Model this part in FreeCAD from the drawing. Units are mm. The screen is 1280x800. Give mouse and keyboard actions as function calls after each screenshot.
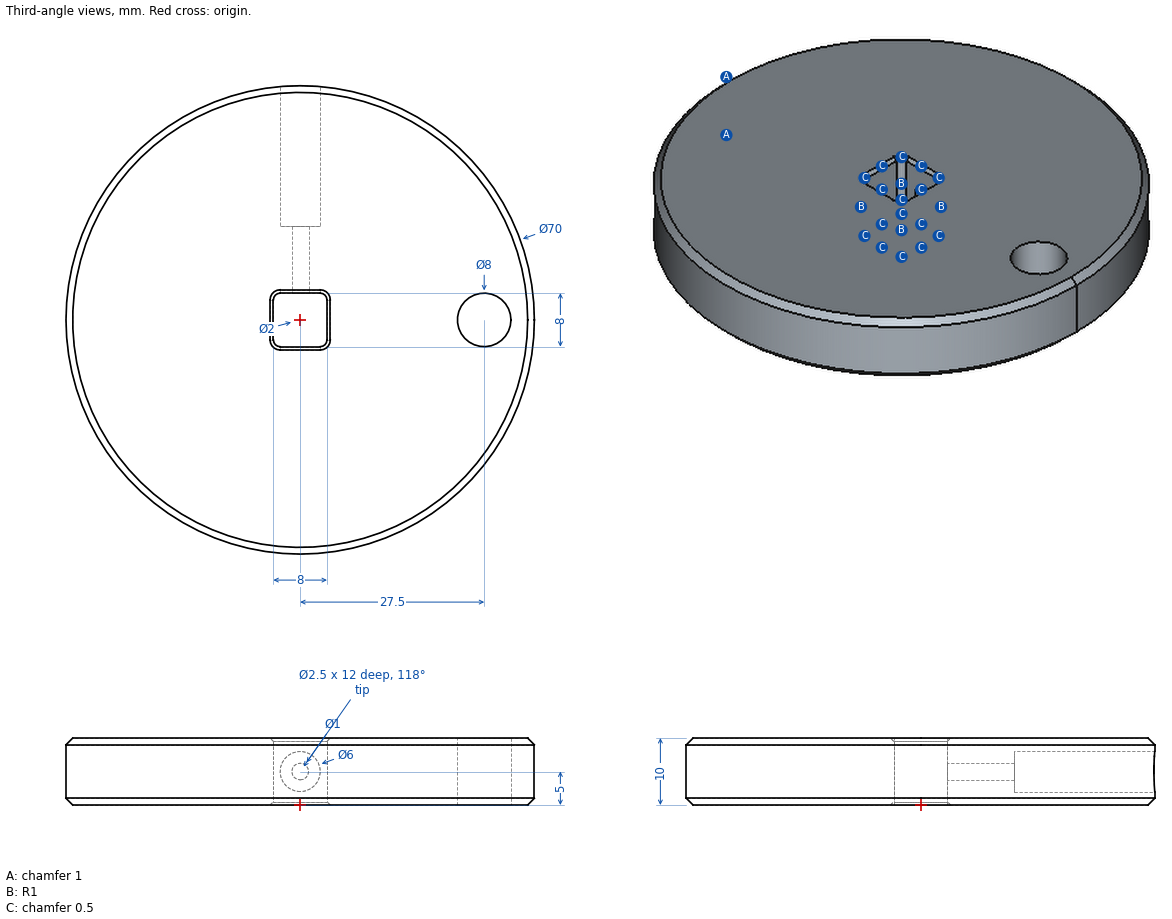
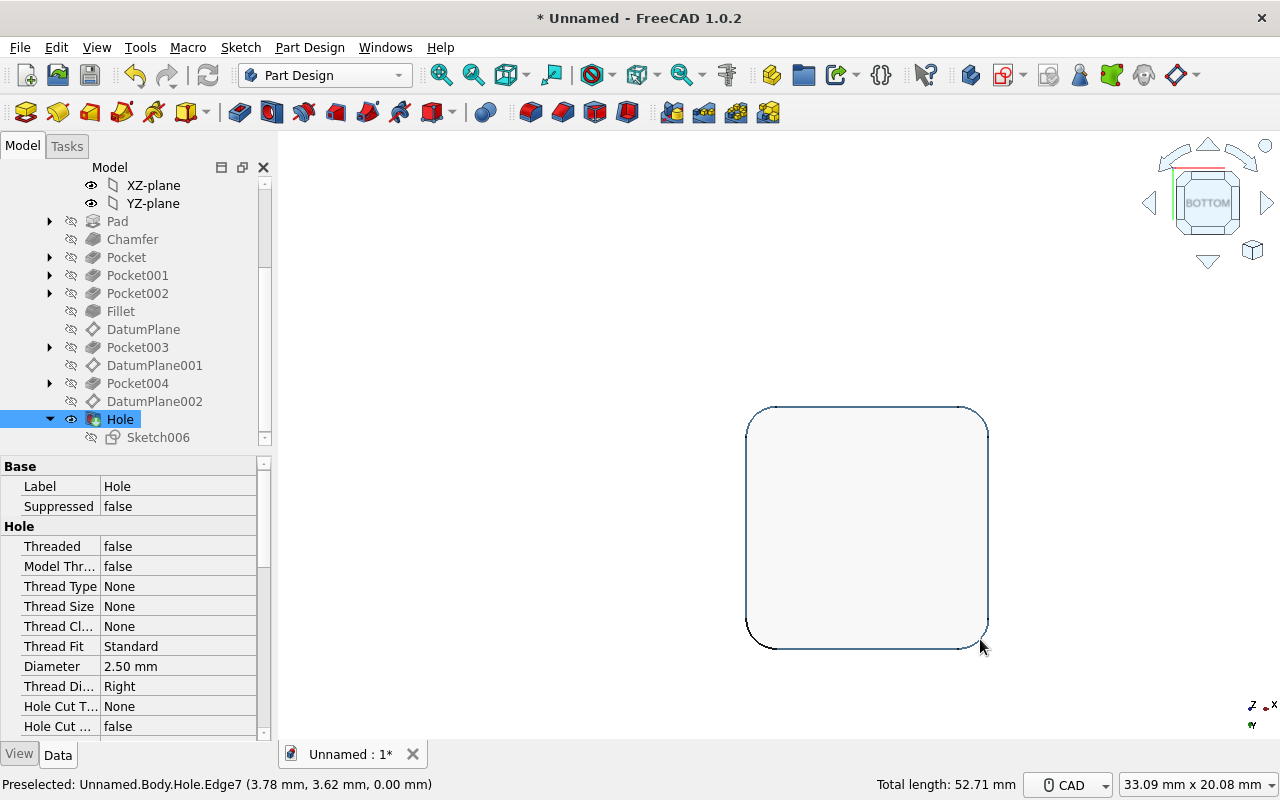
click(759, 642, ctrl)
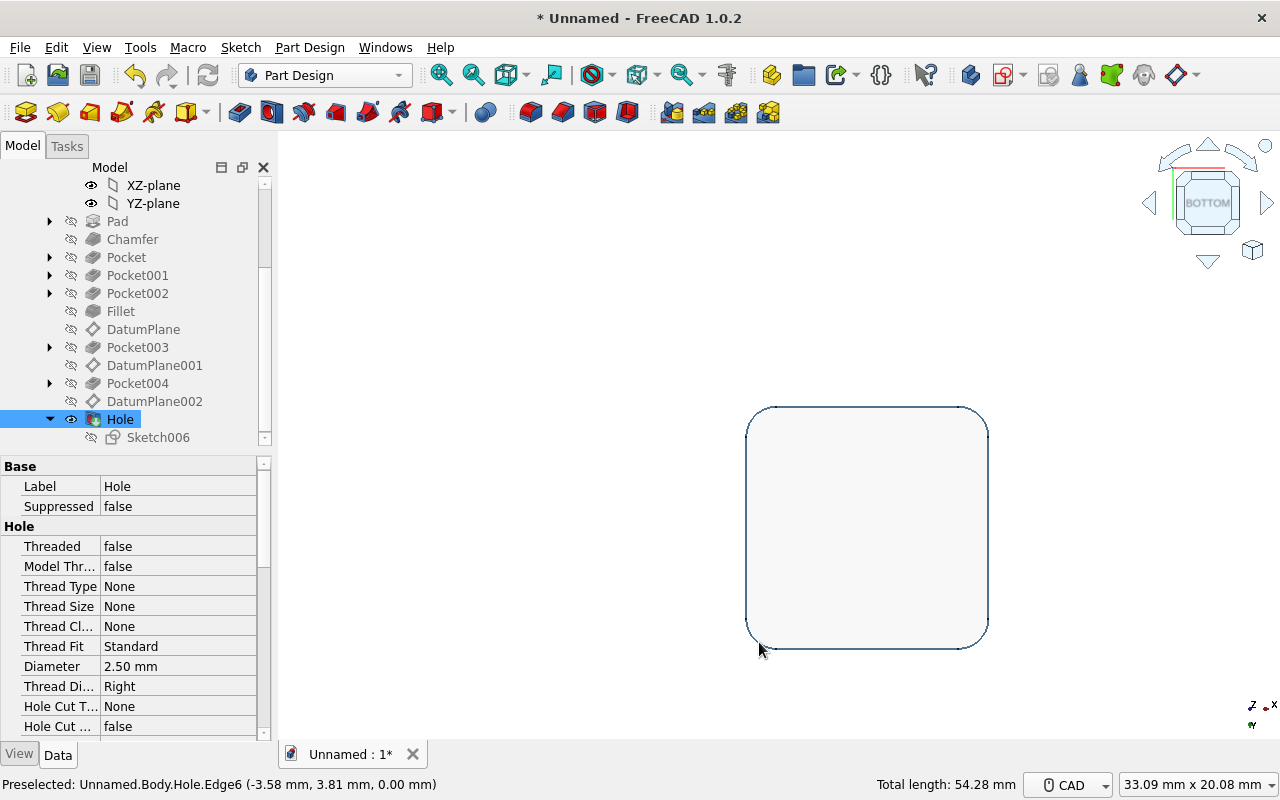
key(v)
key(f)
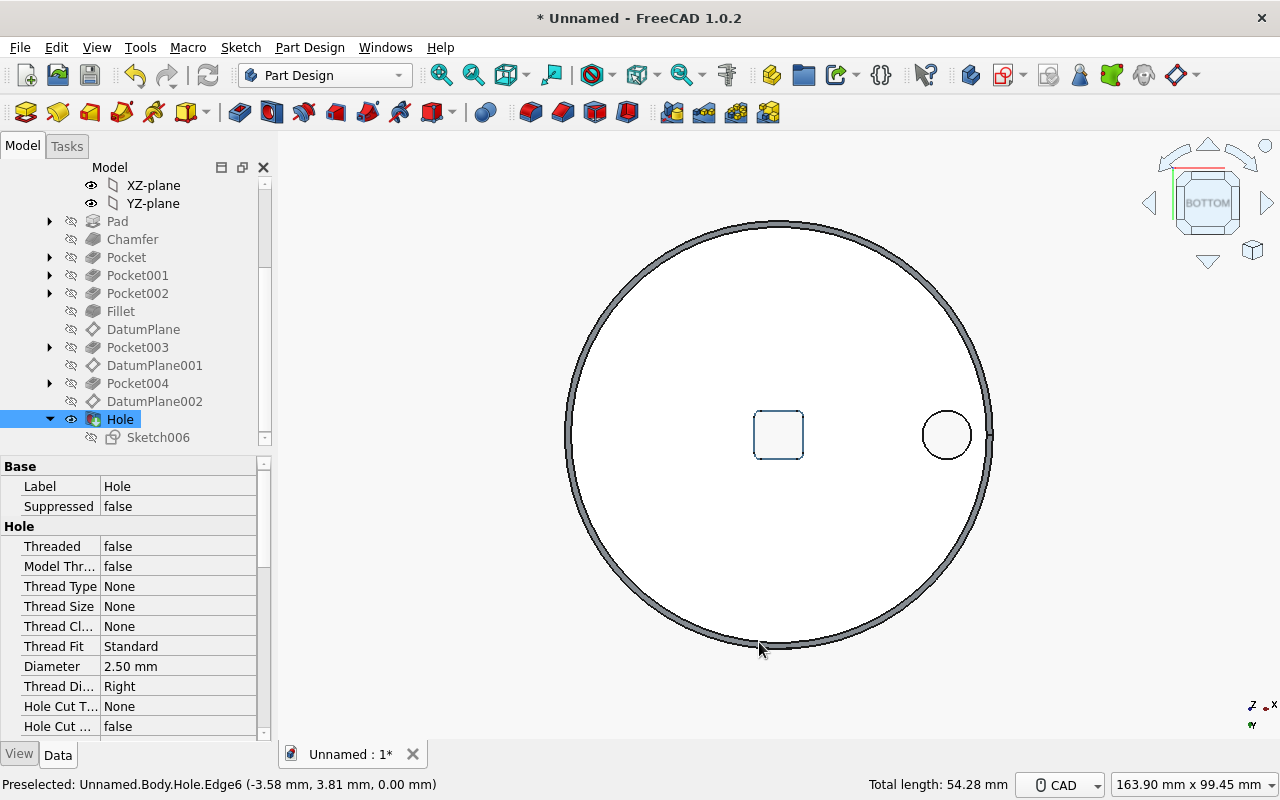
key(4)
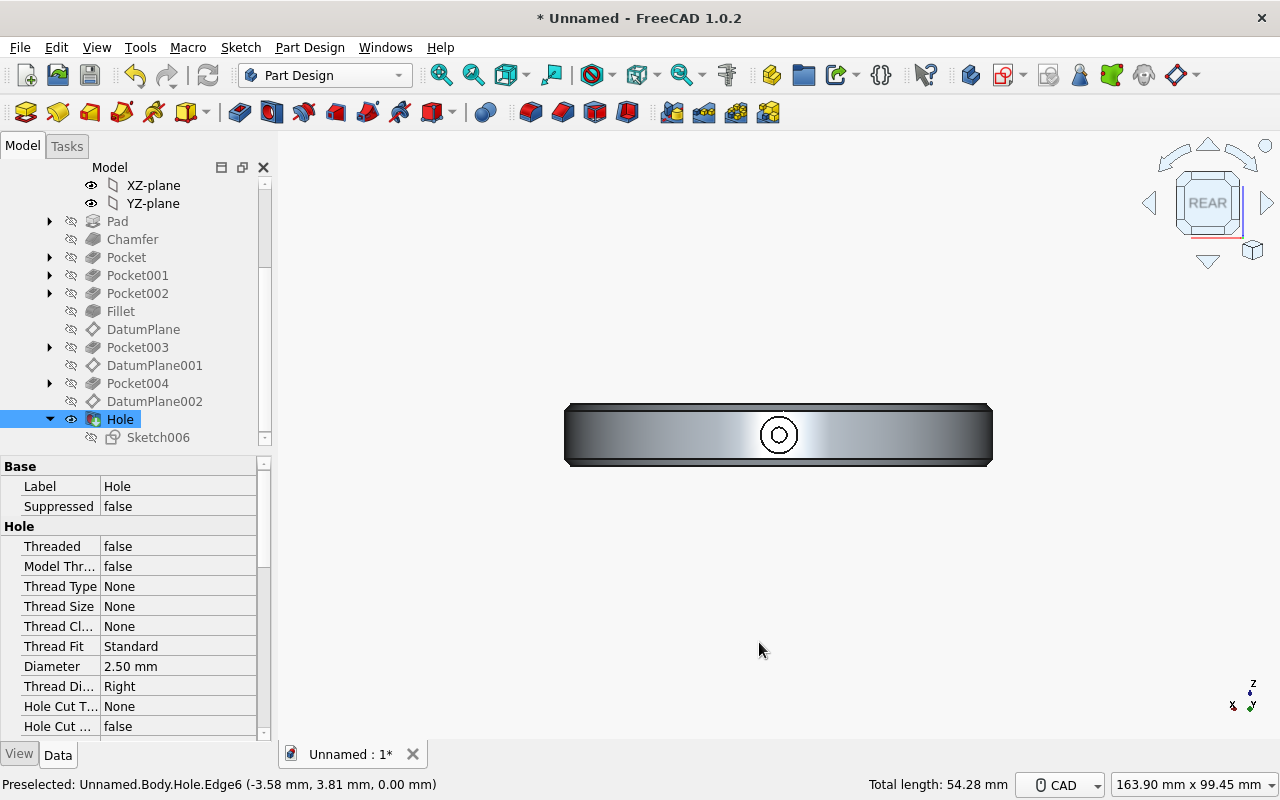
key(v)
key(f)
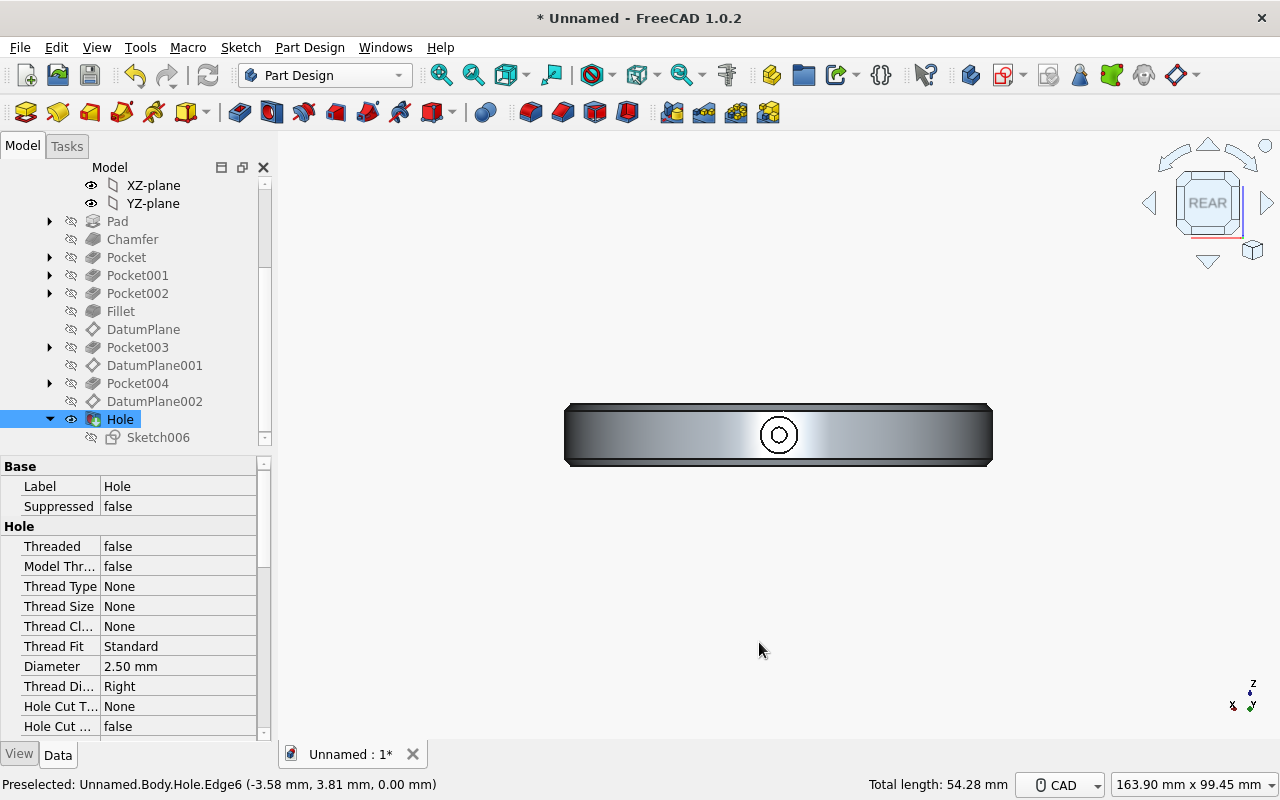
scroll(802, 403, up, 8)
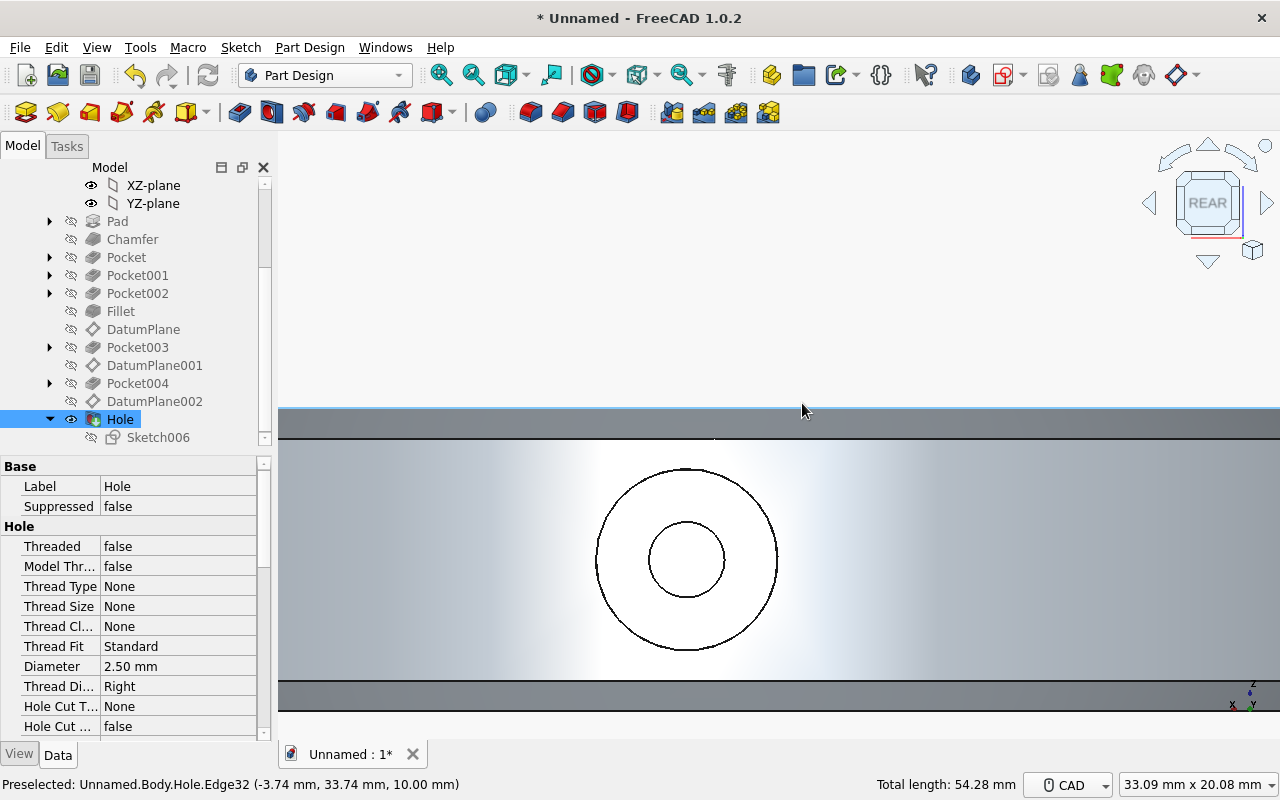
click(442, 76)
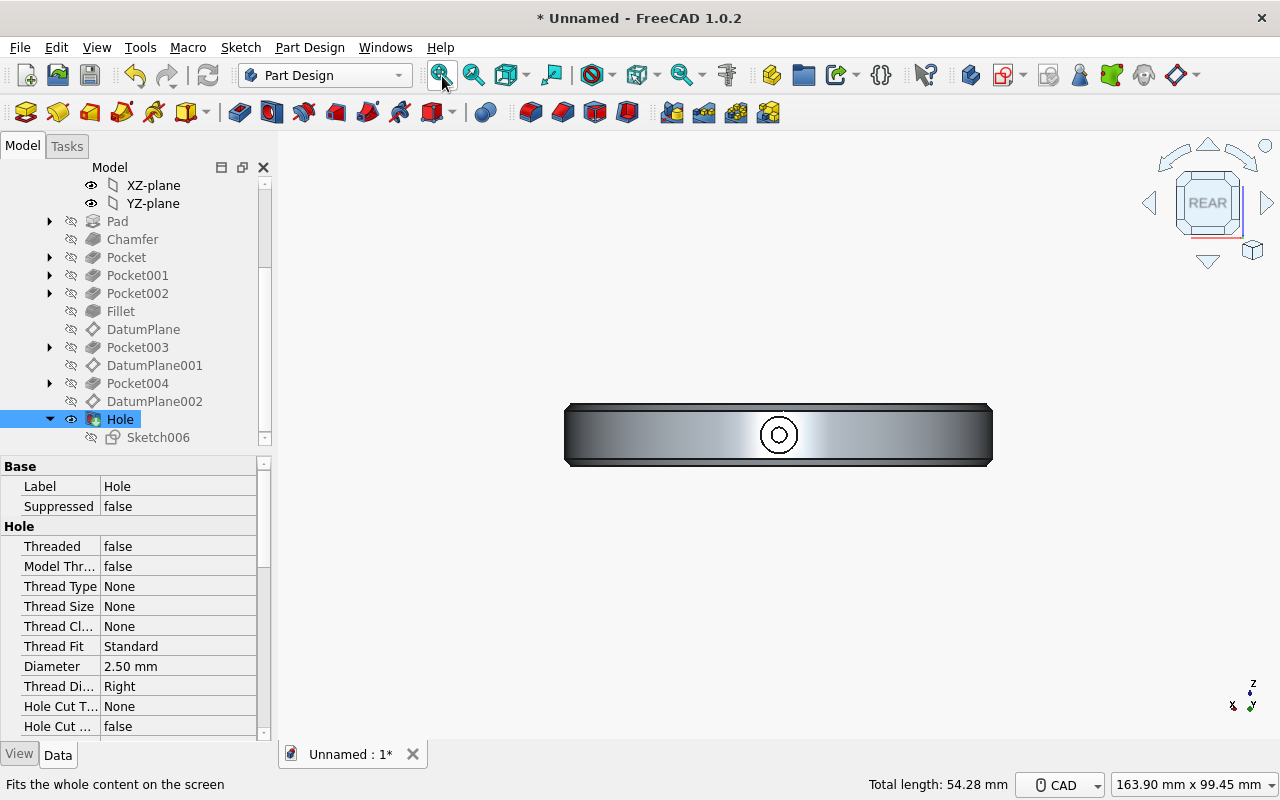
key(6)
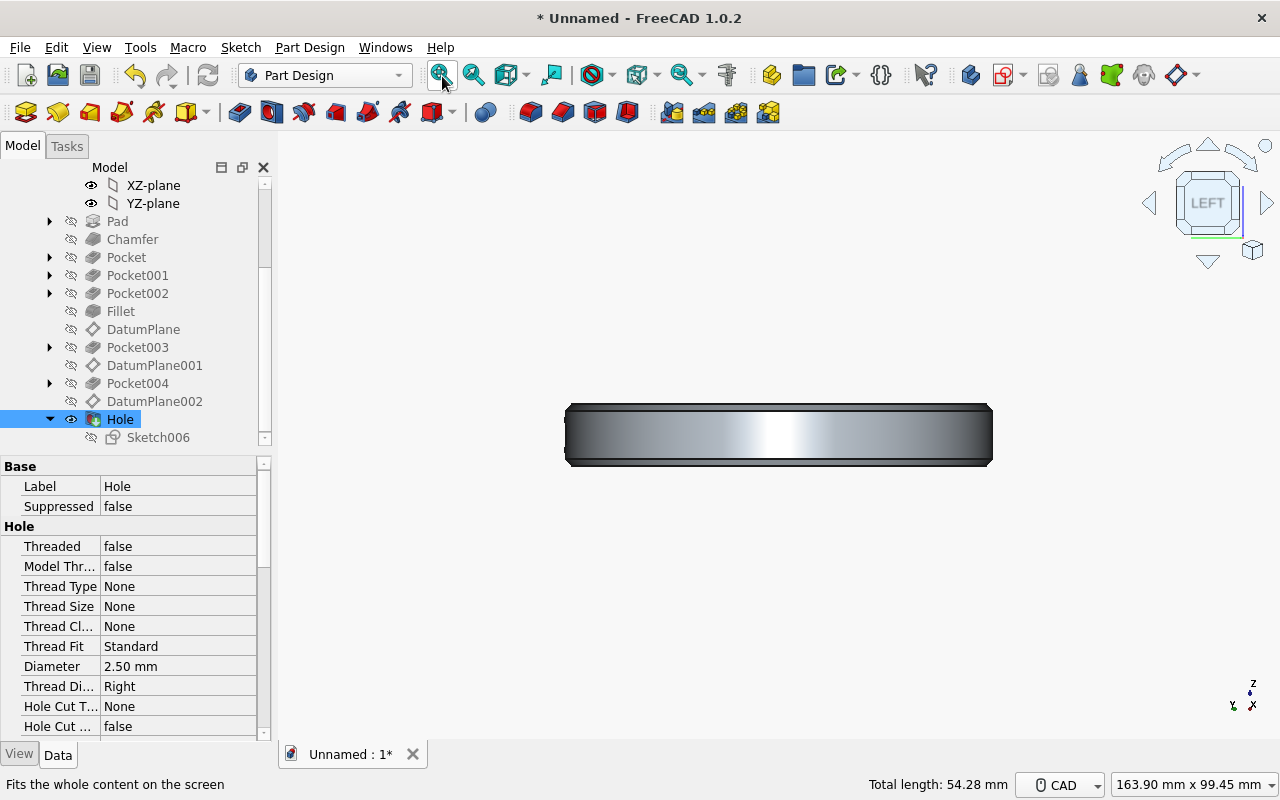
key(v)
key(f)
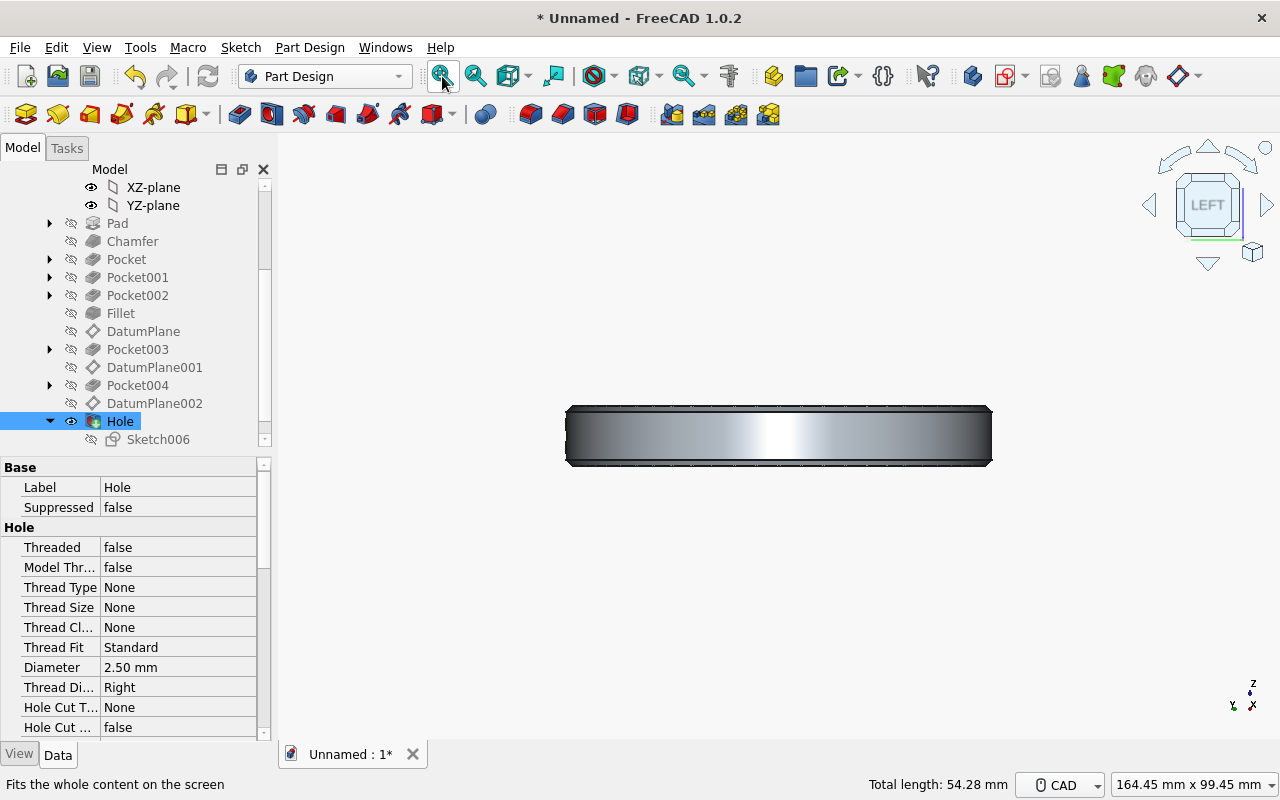
scroll(802, 405, up, 8)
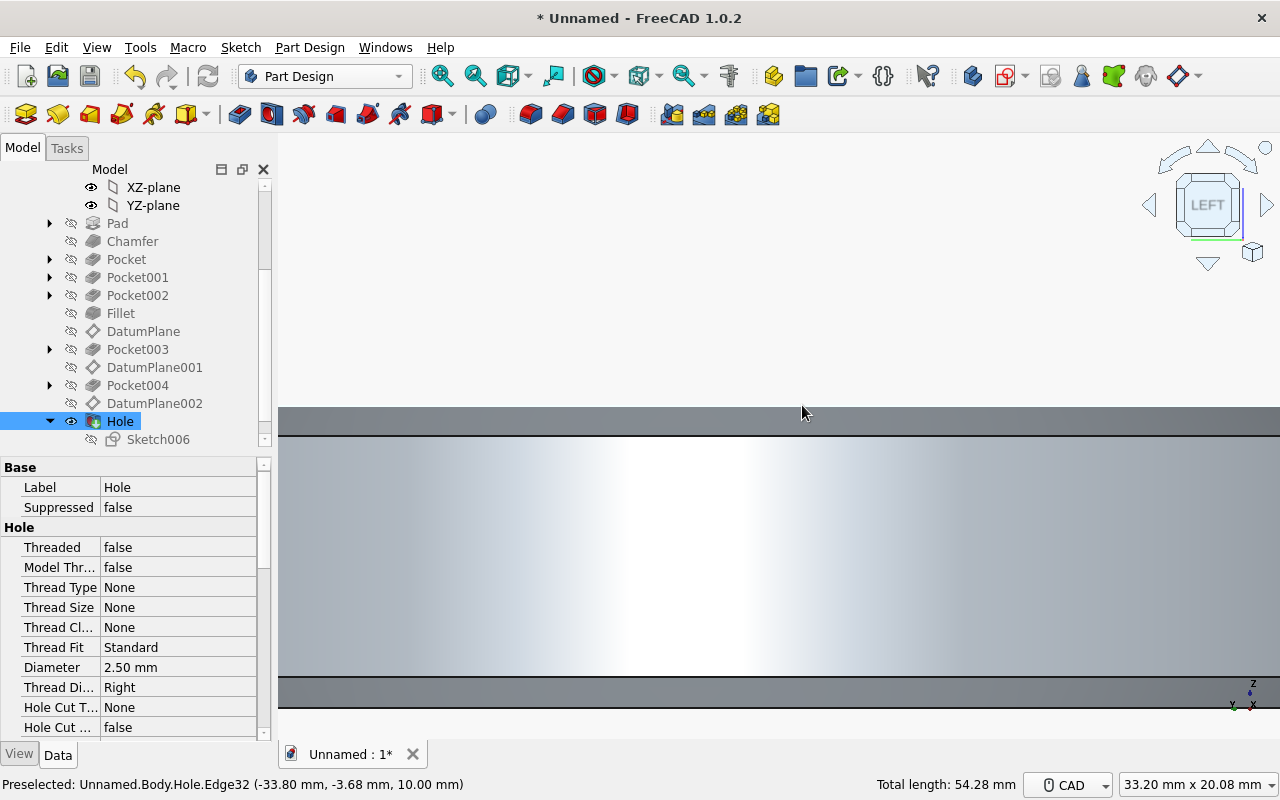
click(444, 76)